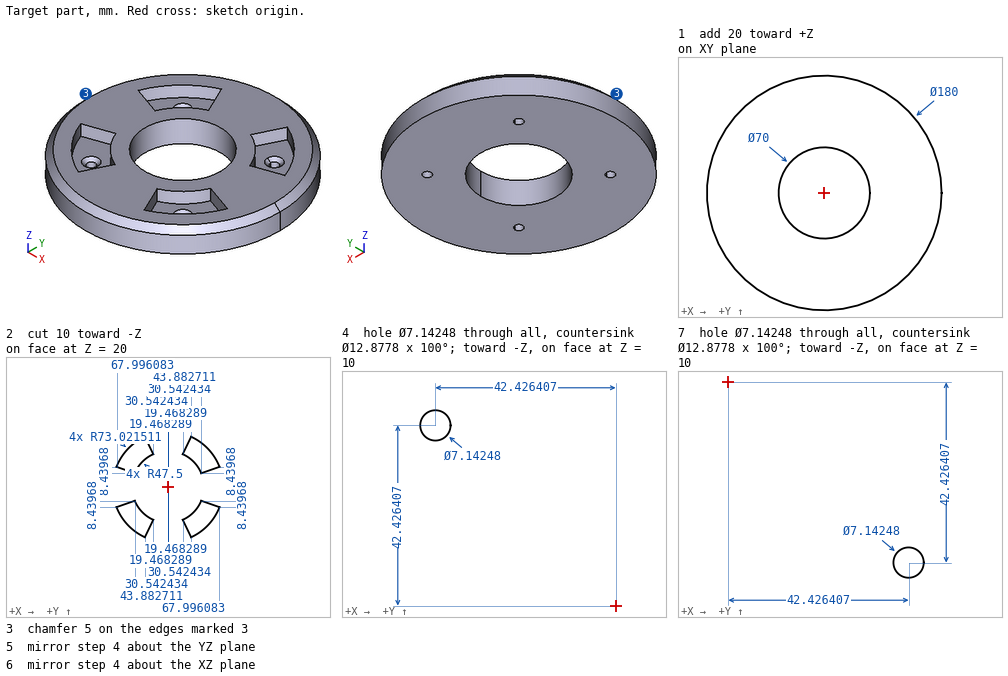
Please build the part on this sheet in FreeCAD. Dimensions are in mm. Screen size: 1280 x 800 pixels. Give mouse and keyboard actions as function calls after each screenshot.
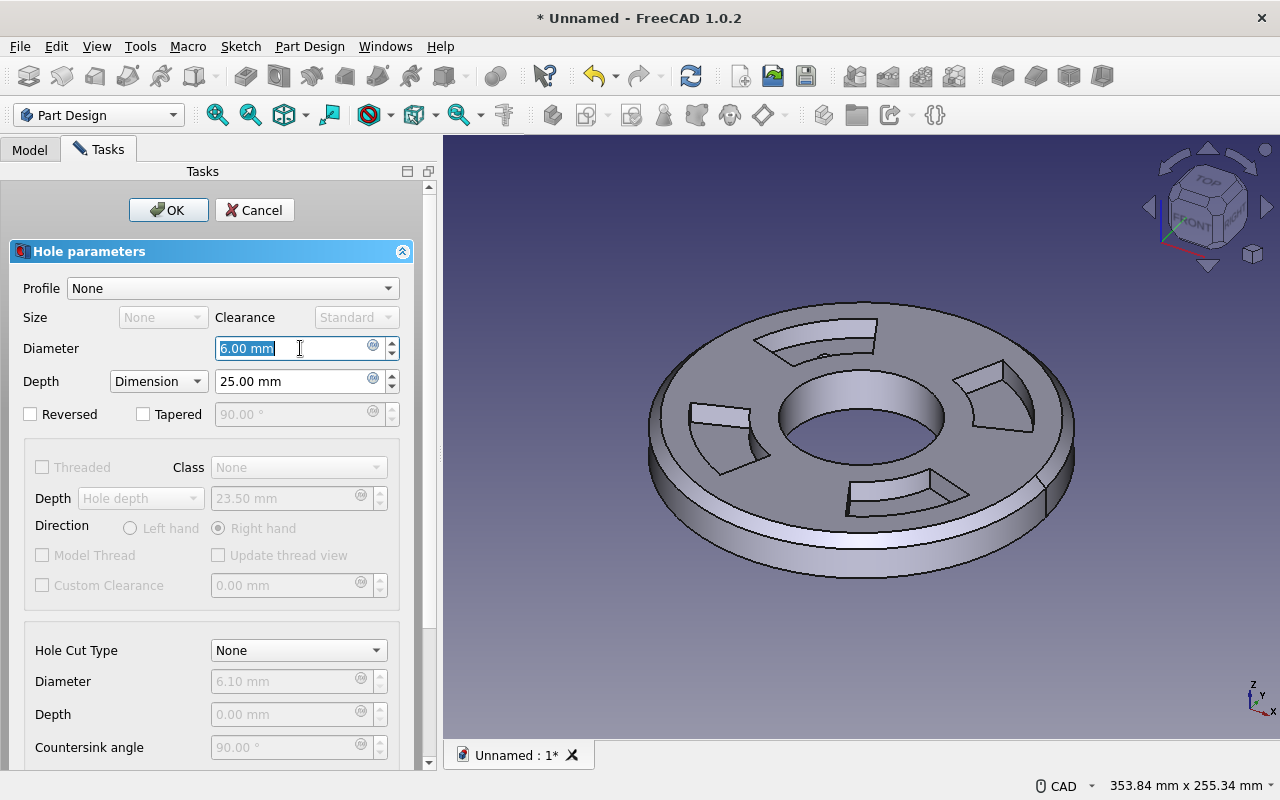
text(7.14248)
key(Tab)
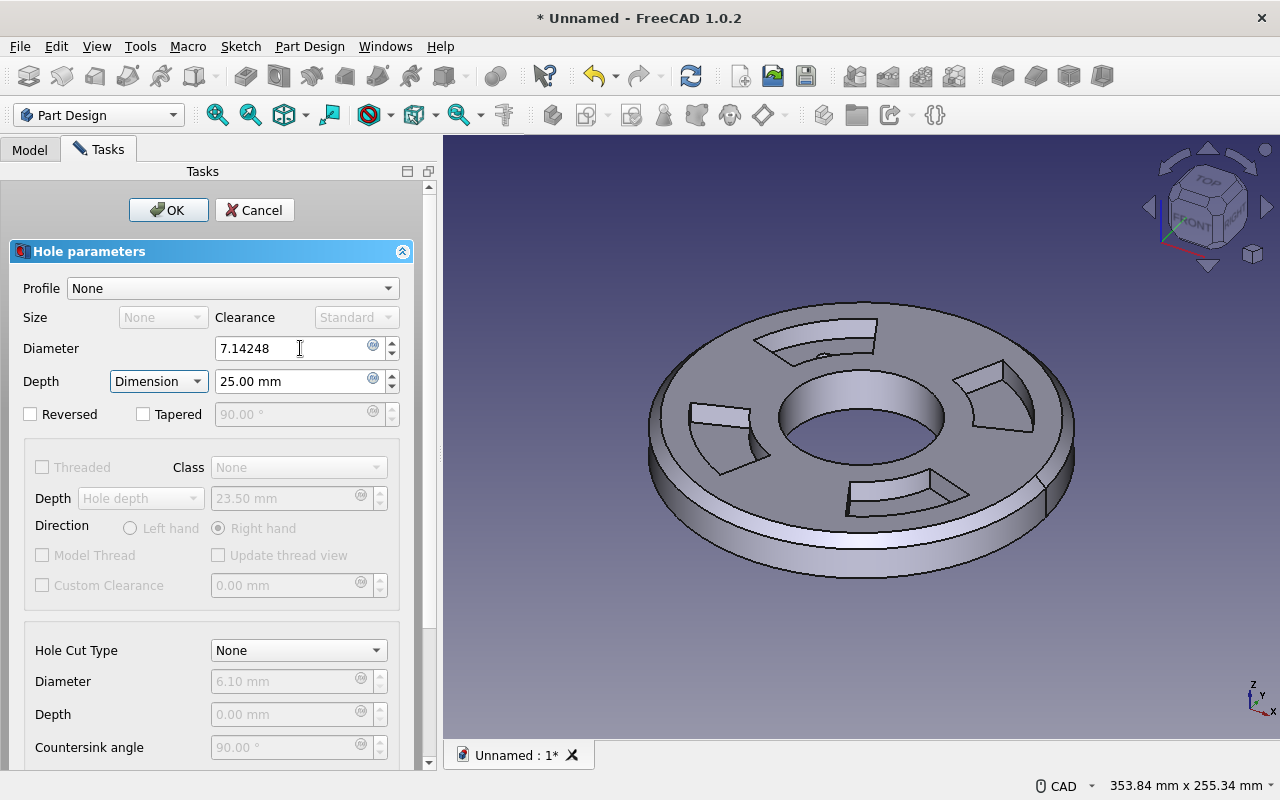
click(160, 382)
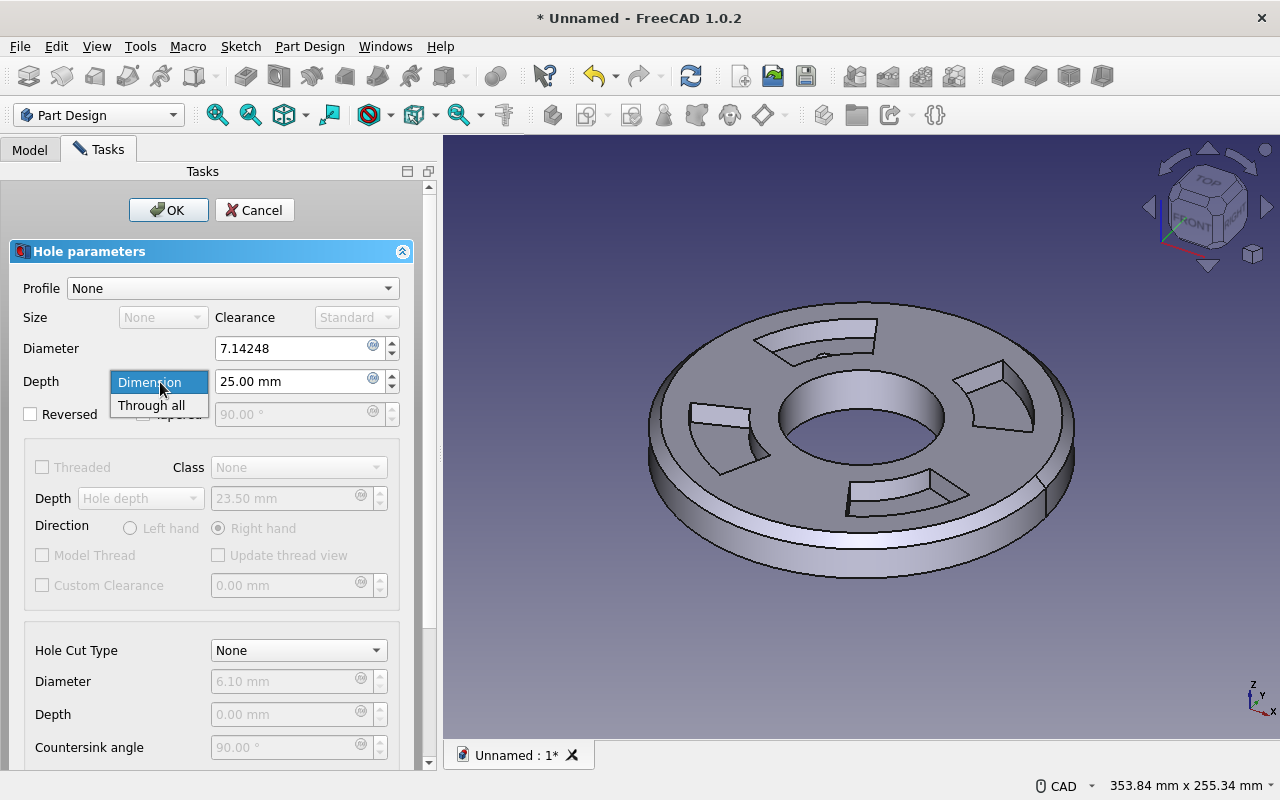
click(158, 406)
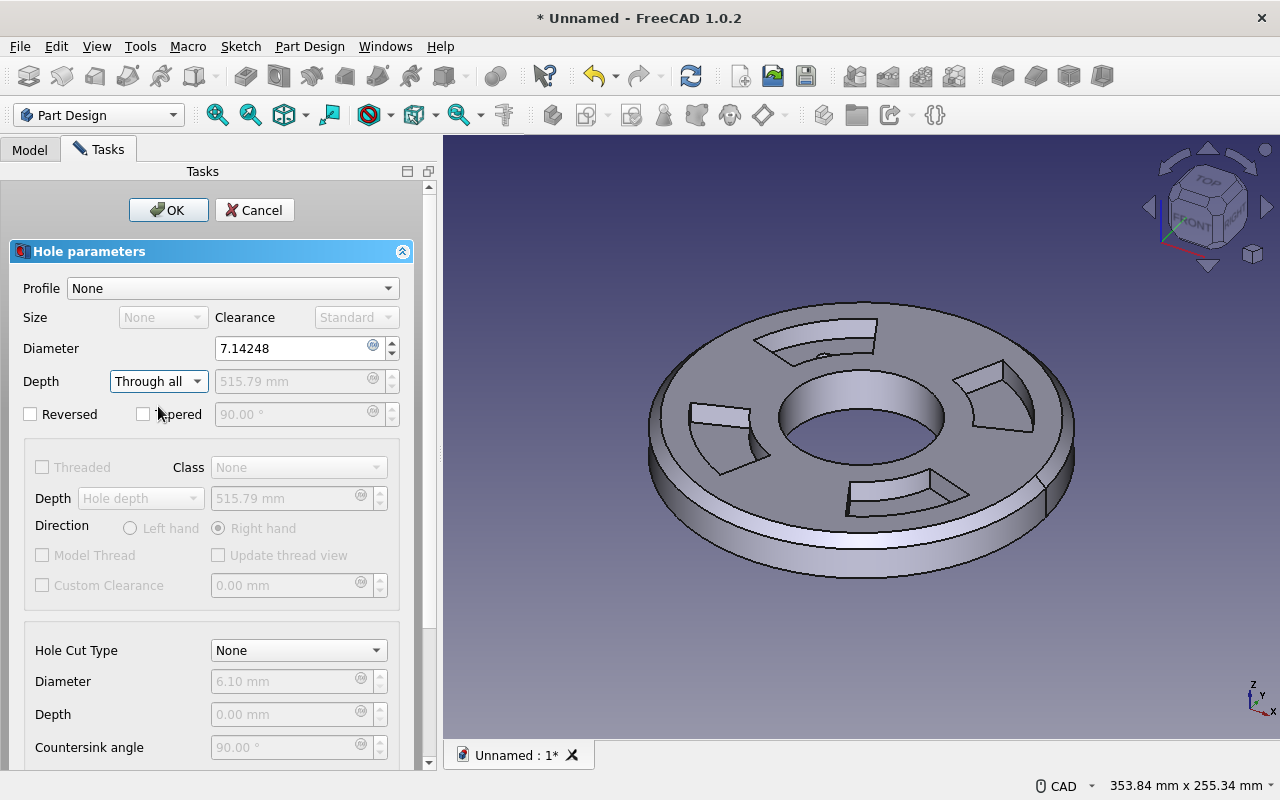
click(300, 650)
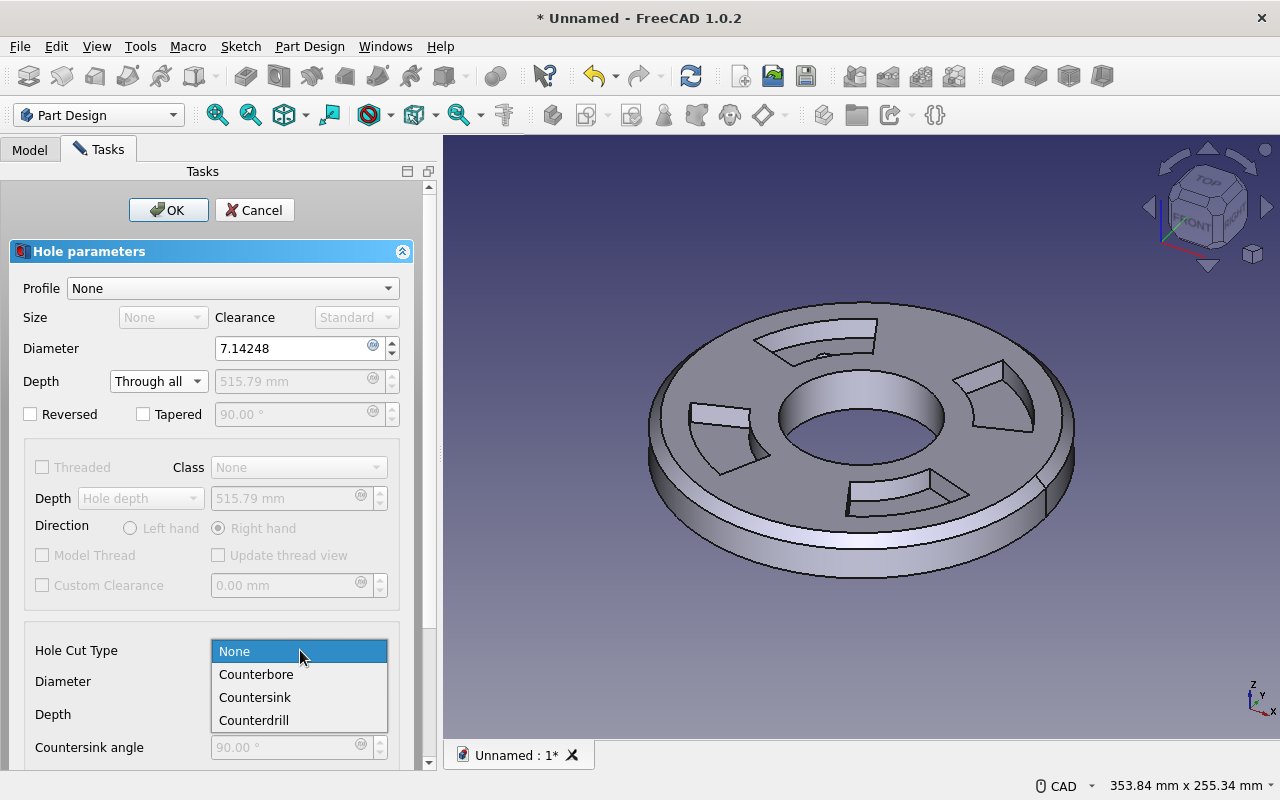
click(298, 698)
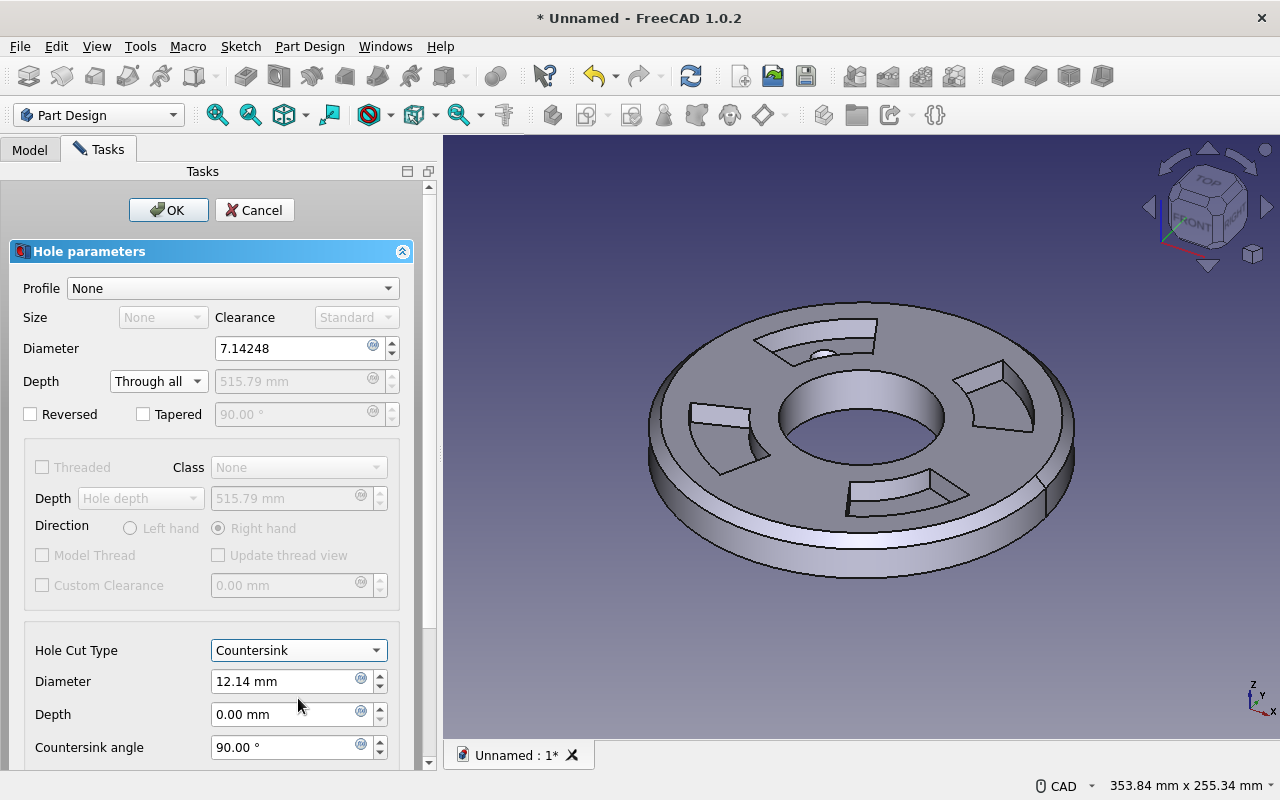
triple_click(292, 748)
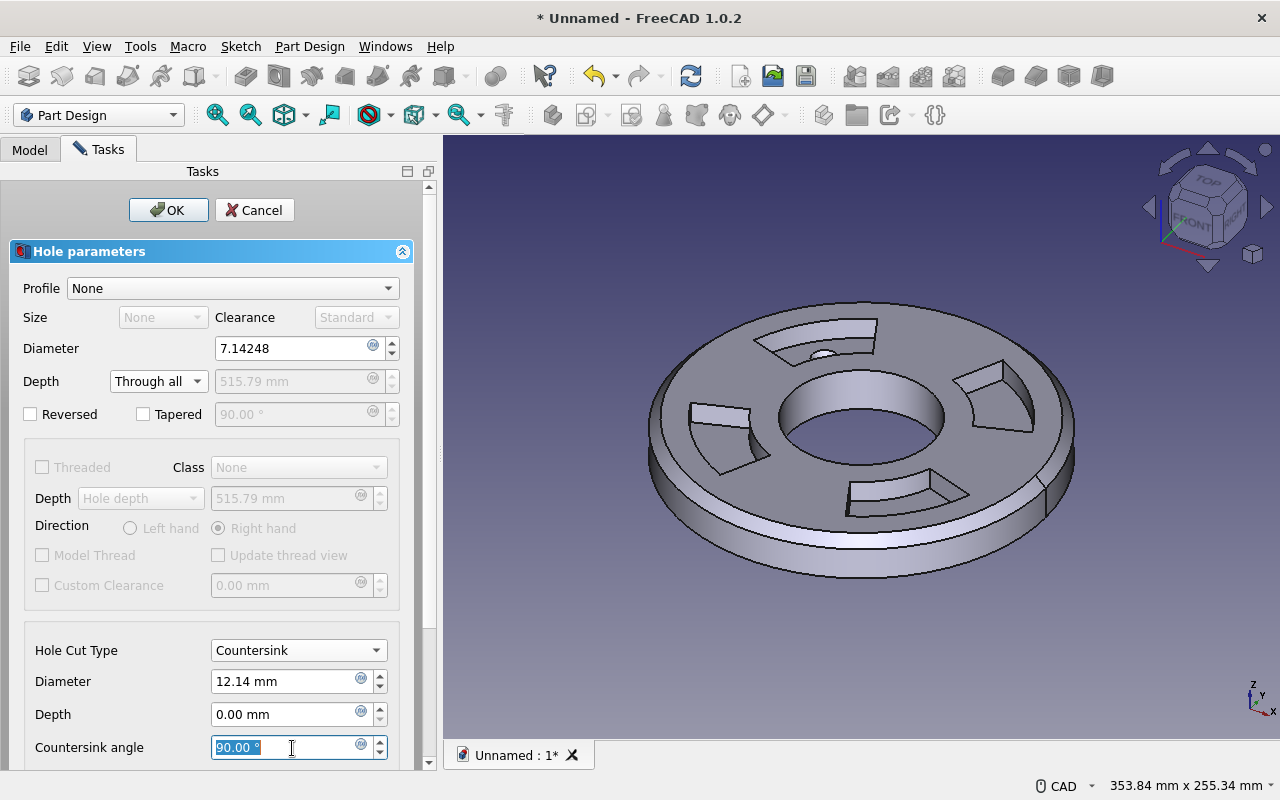
text(100)
key(Tab)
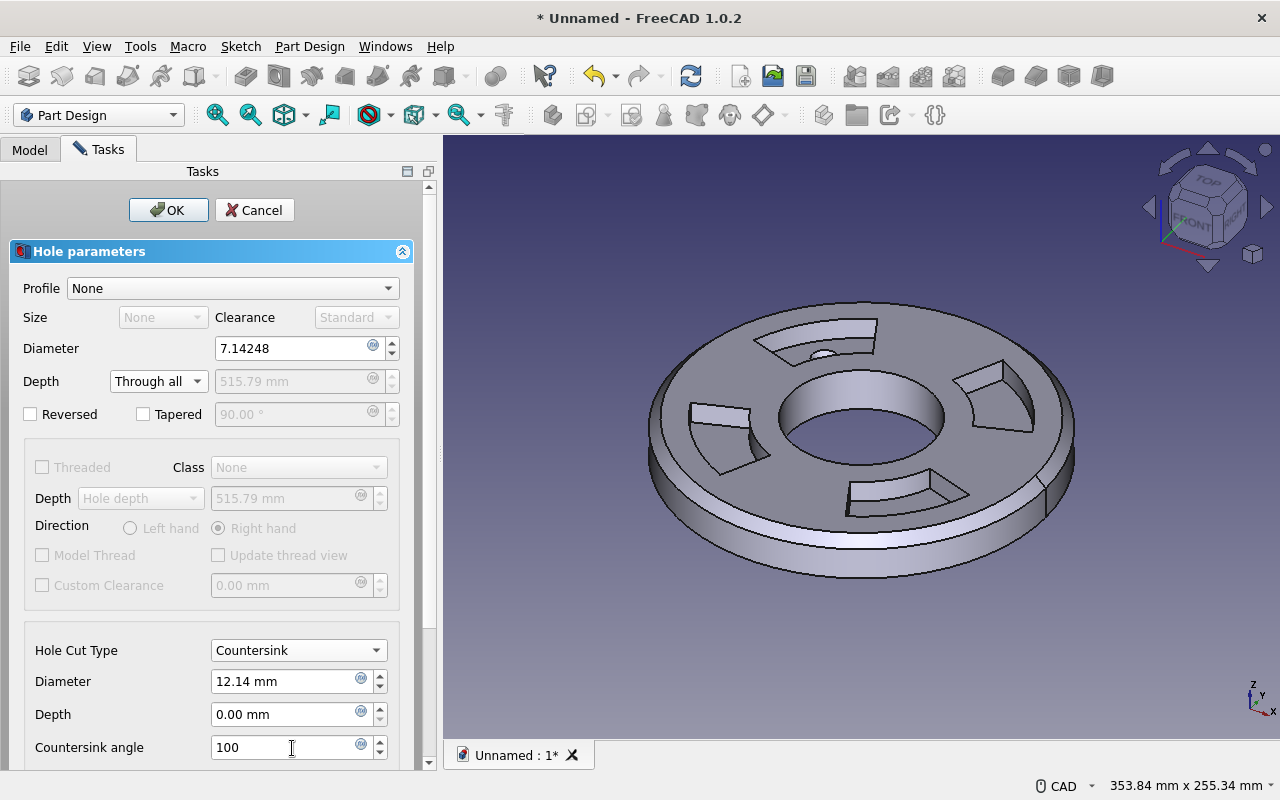
triple_click(292, 682)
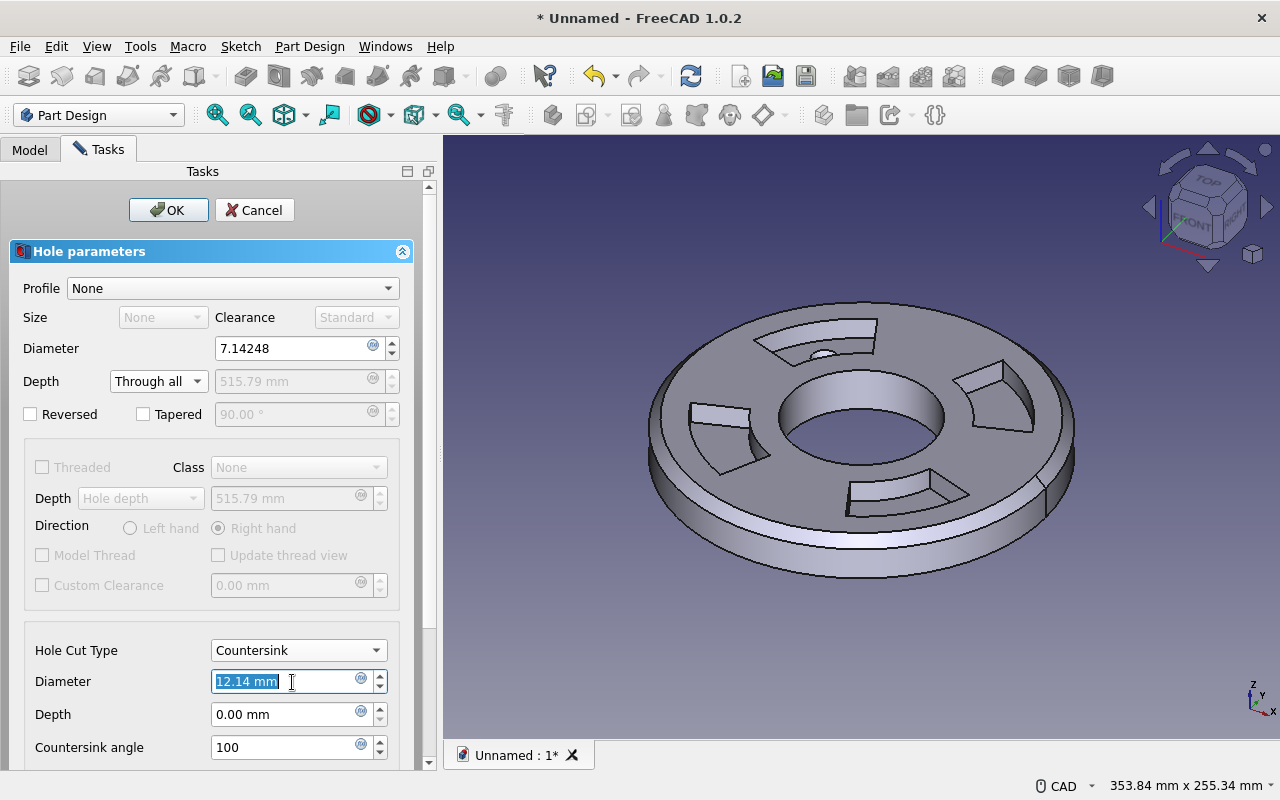
text(12.8778)
key(Tab)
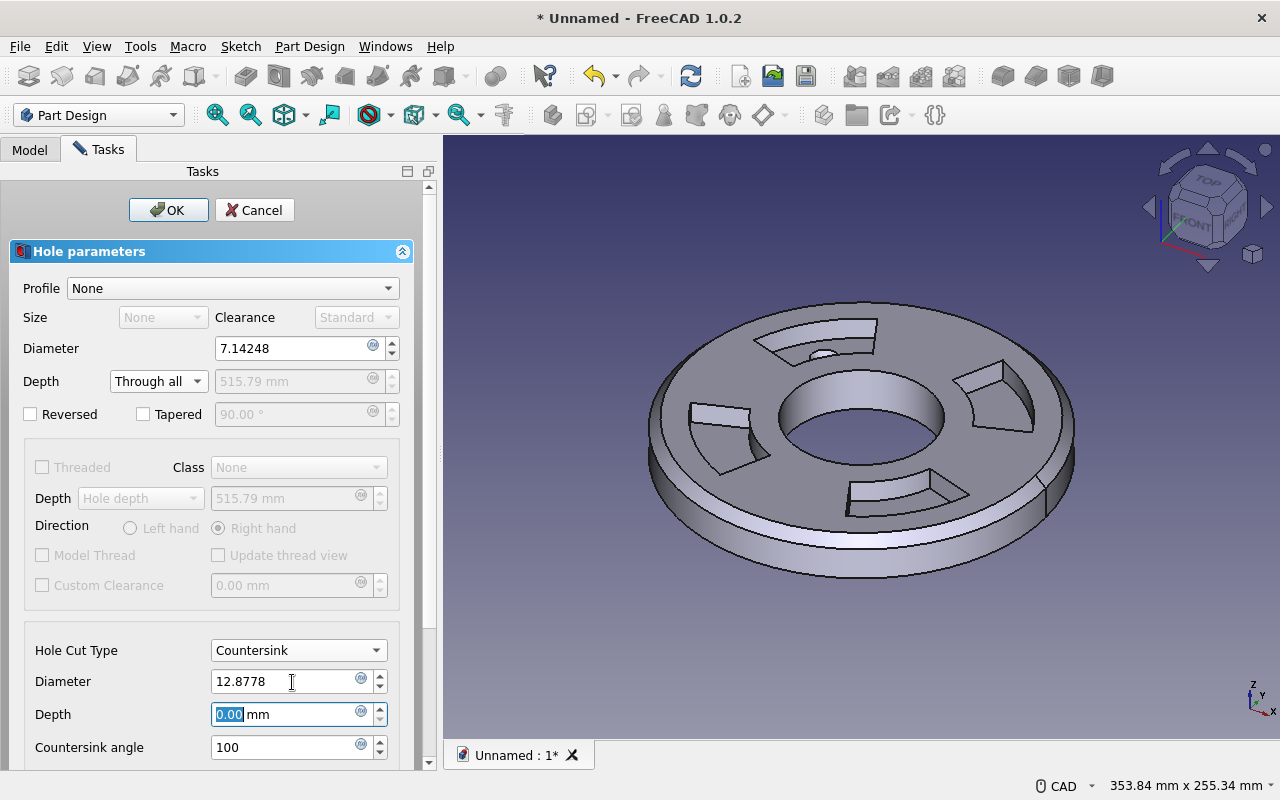
click(169, 210)